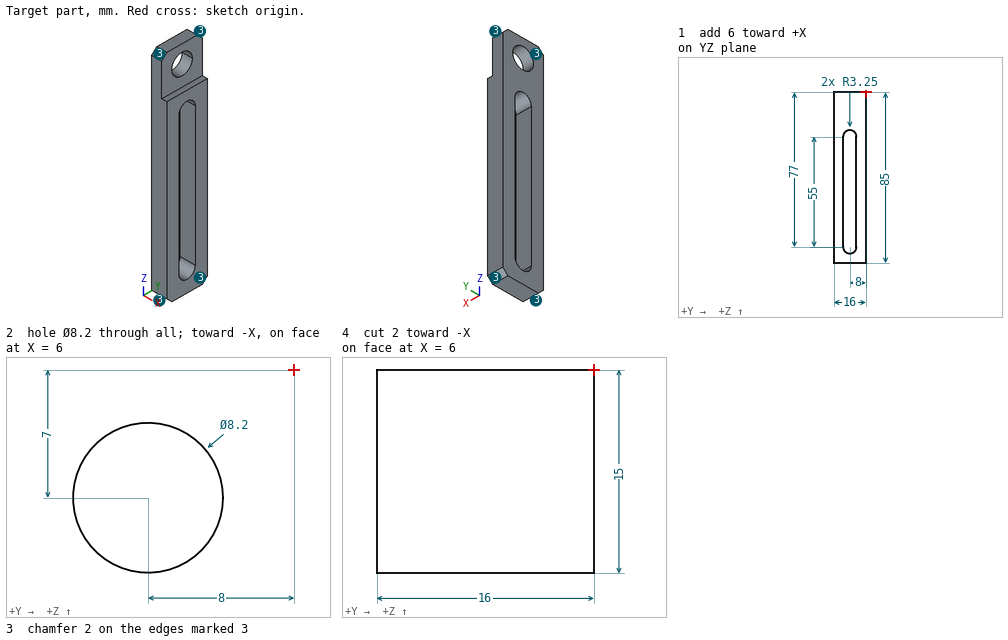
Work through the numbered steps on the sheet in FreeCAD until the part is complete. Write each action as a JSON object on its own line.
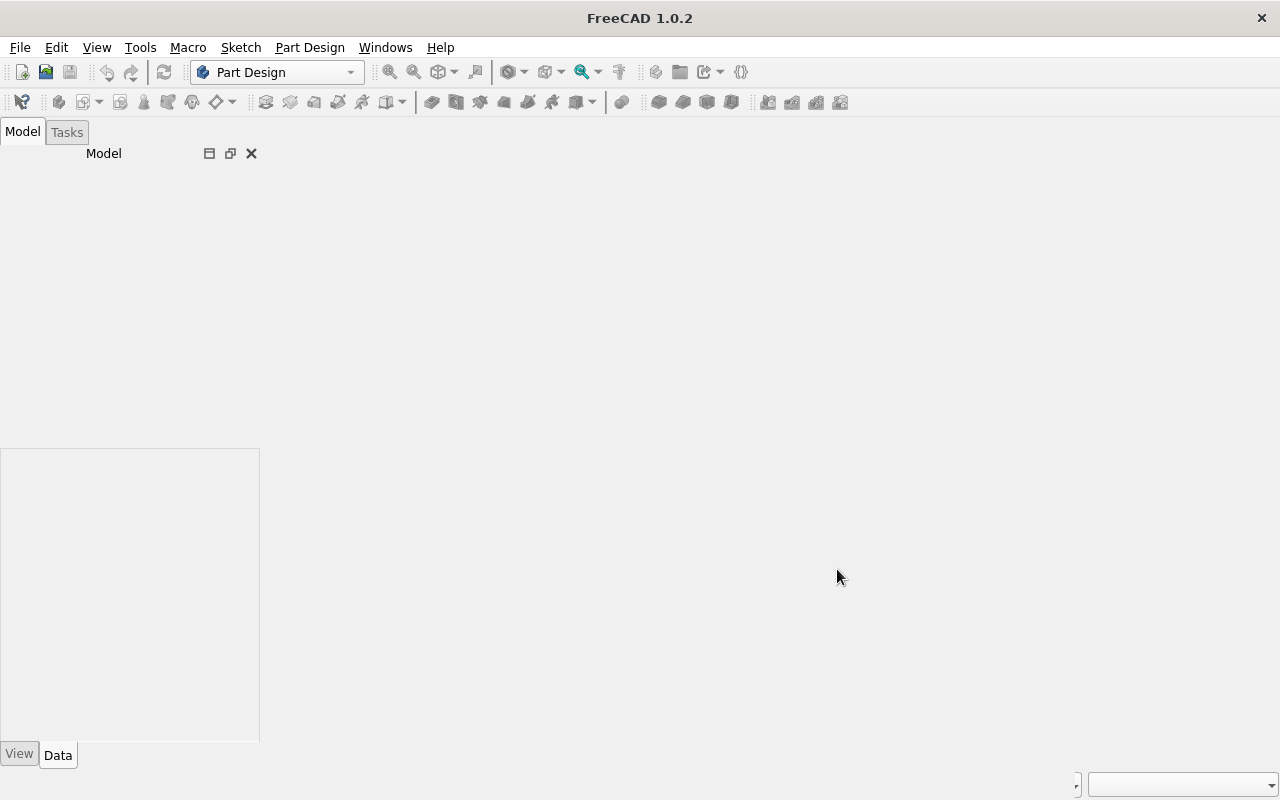
{"action": "key", "text": "ctrl+n"}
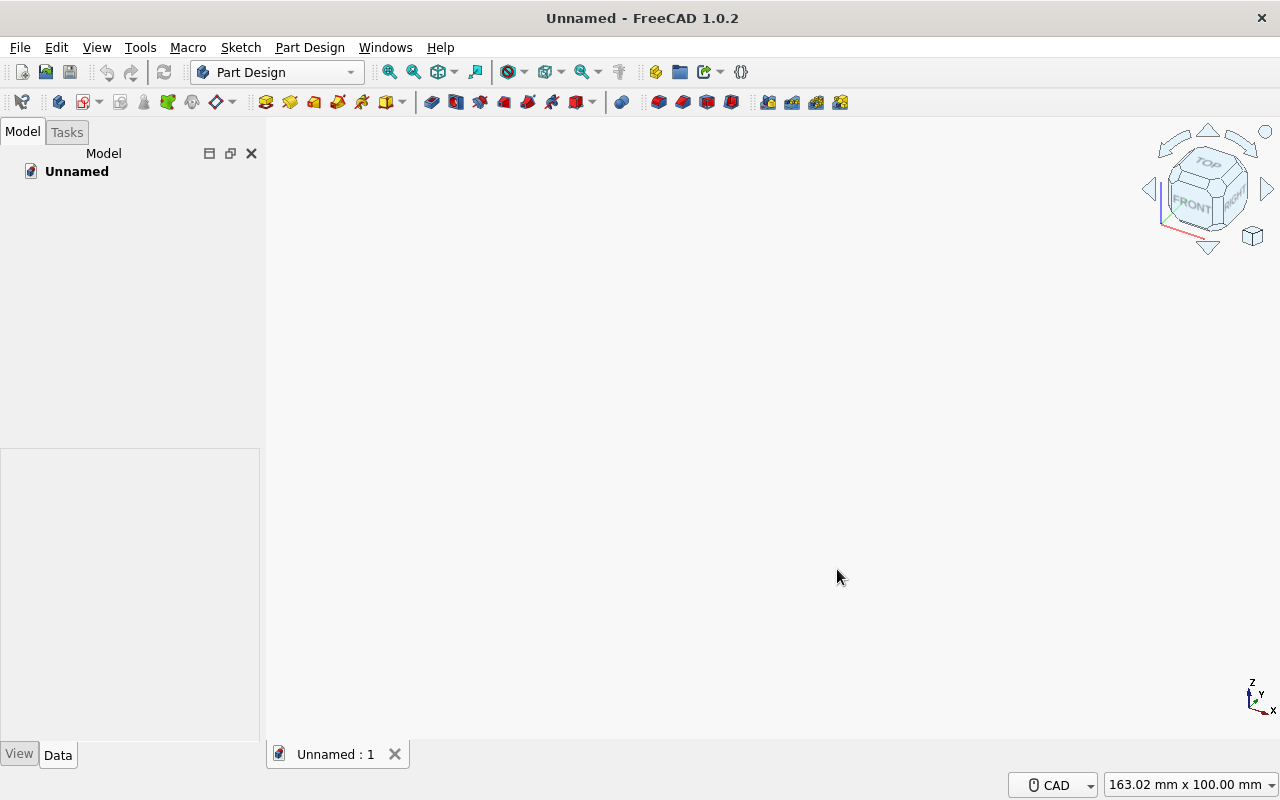
{"action": "left_click", "coordinate": [84, 102]}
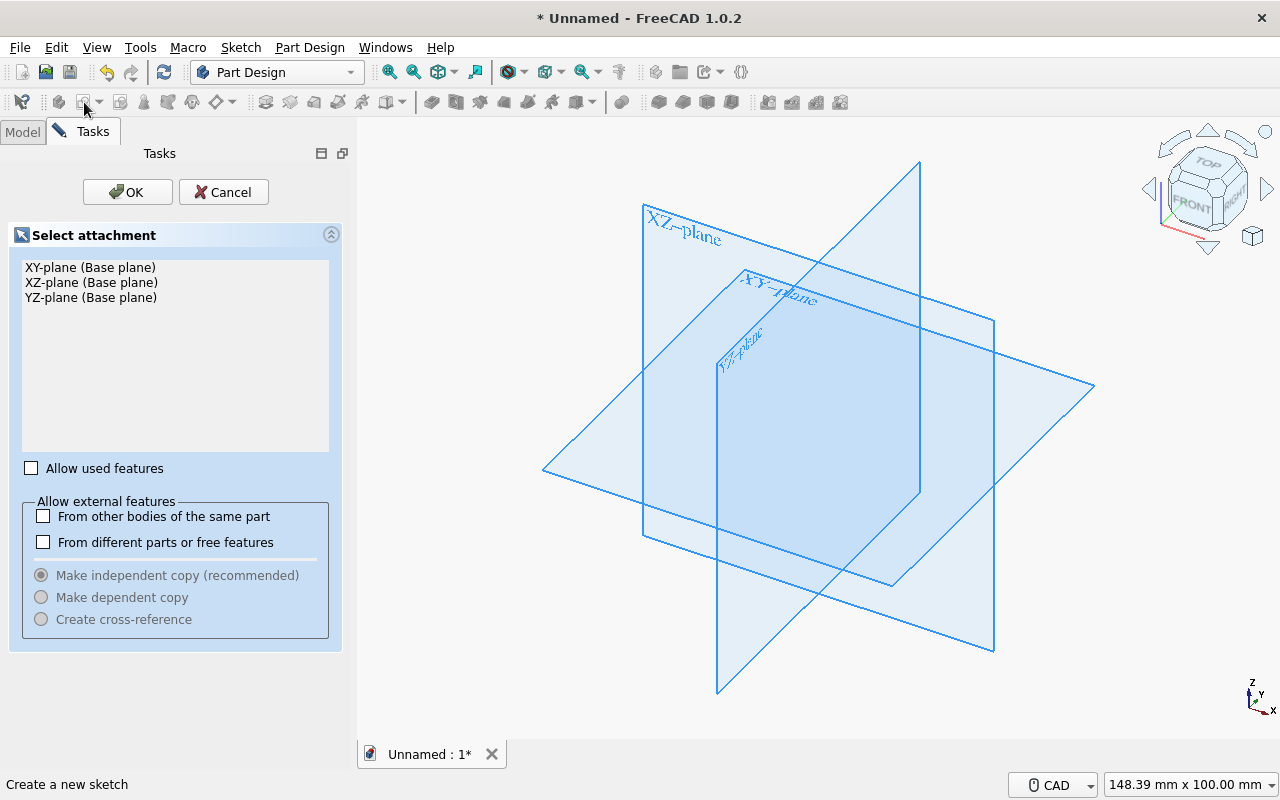
{"action": "left_click", "coordinate": [82, 298]}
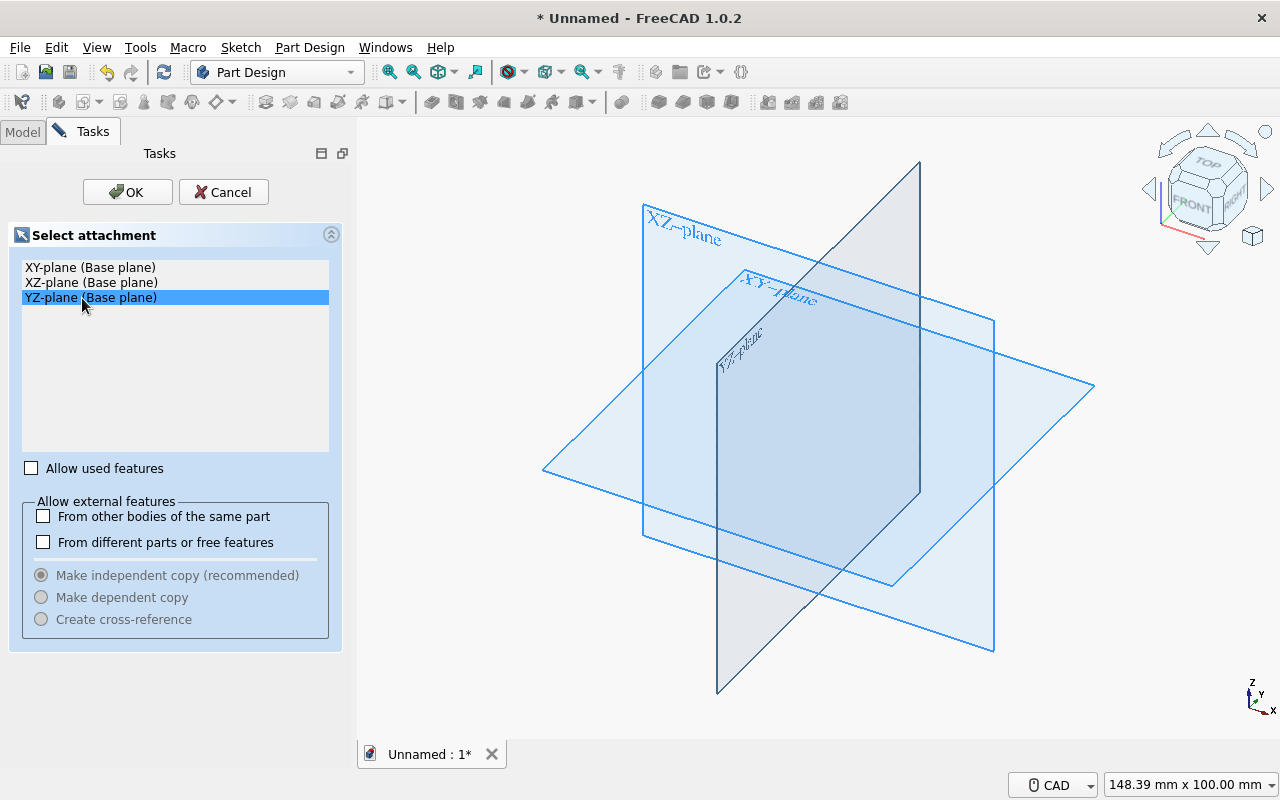
{"action": "left_click", "coordinate": [128, 192]}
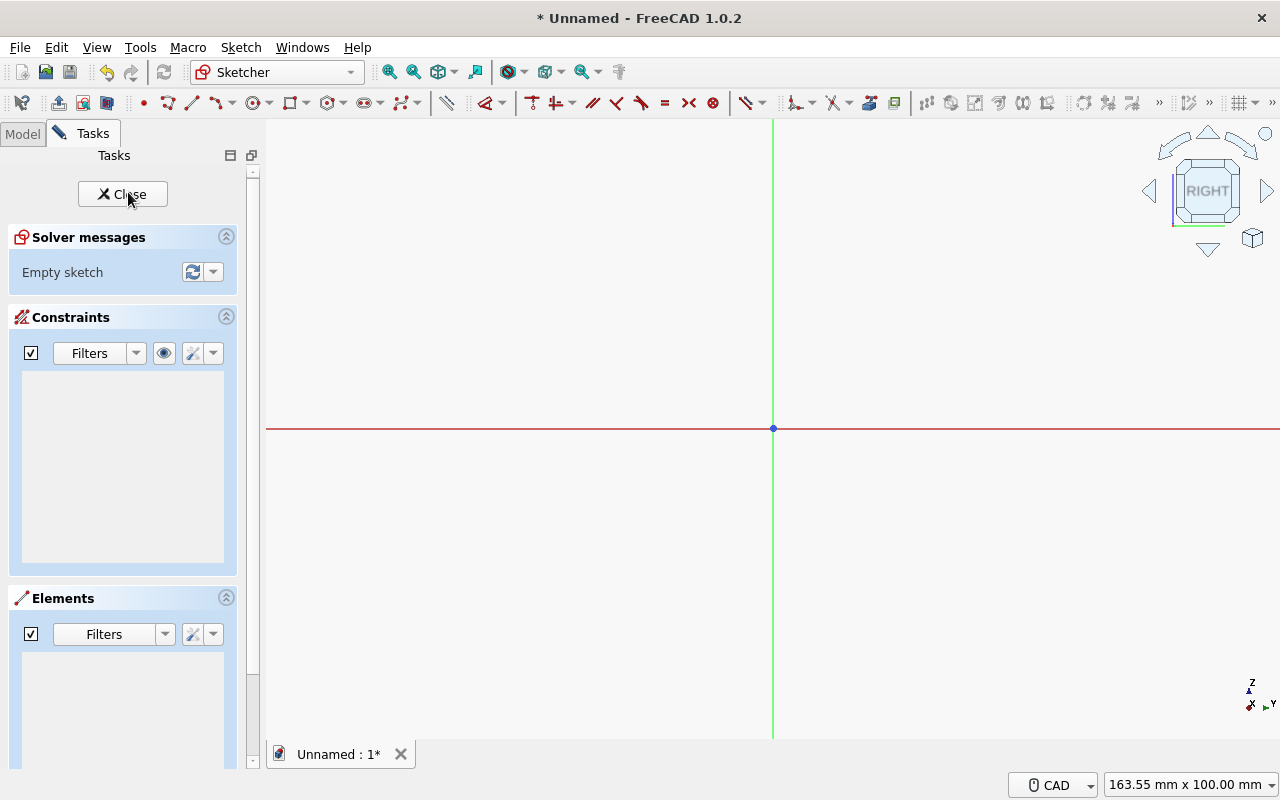
{"action": "scroll", "coordinate": [682, 147], "scroll_direction": "down", "scroll_amount": 3}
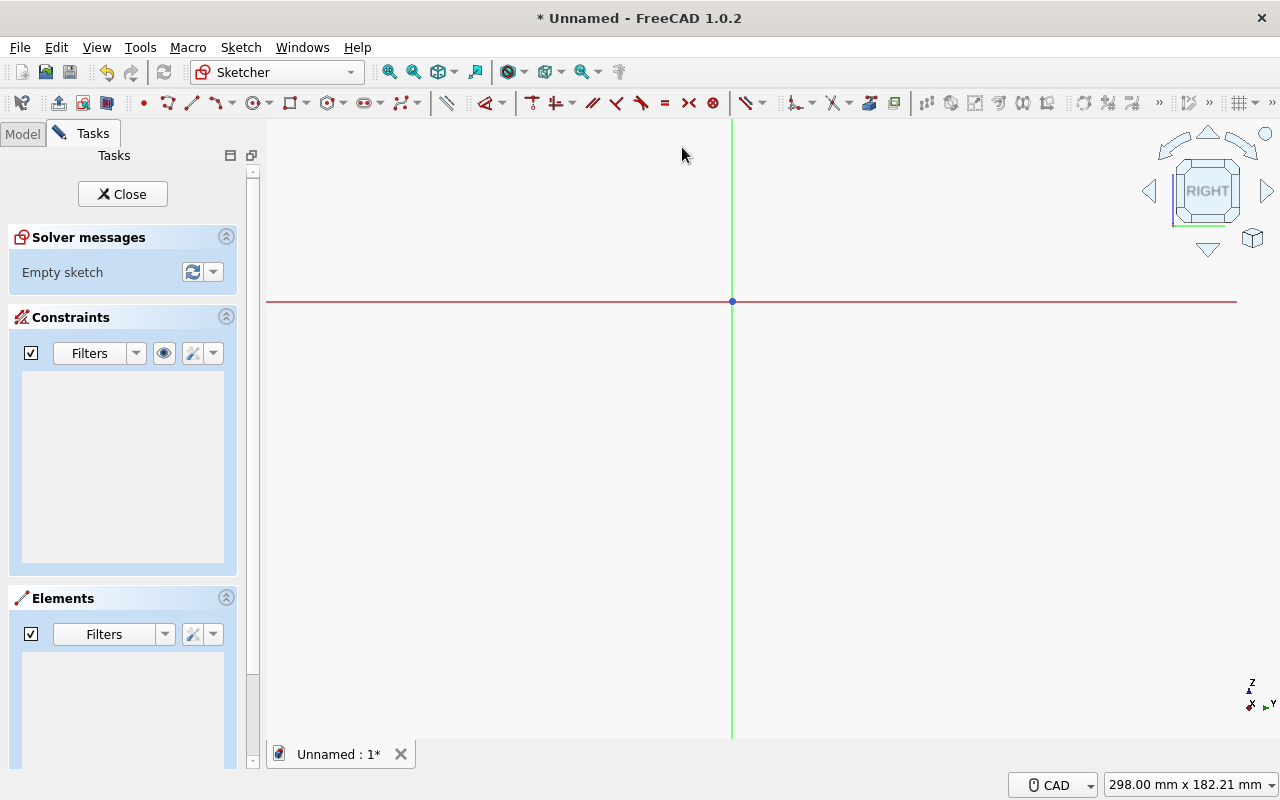
{"action": "scroll", "coordinate": [706, 482], "scroll_direction": "up", "scroll_amount": 2}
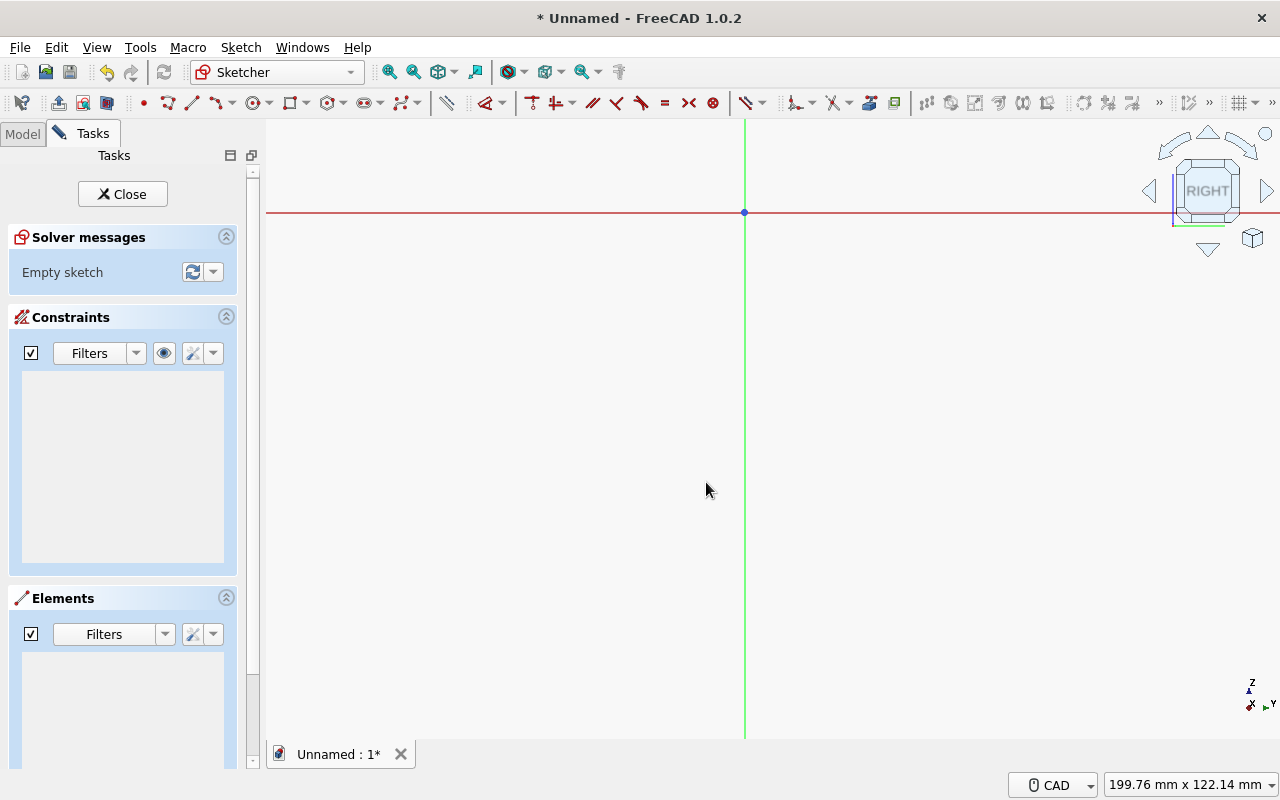
{"action": "left_click", "coordinate": [290, 104]}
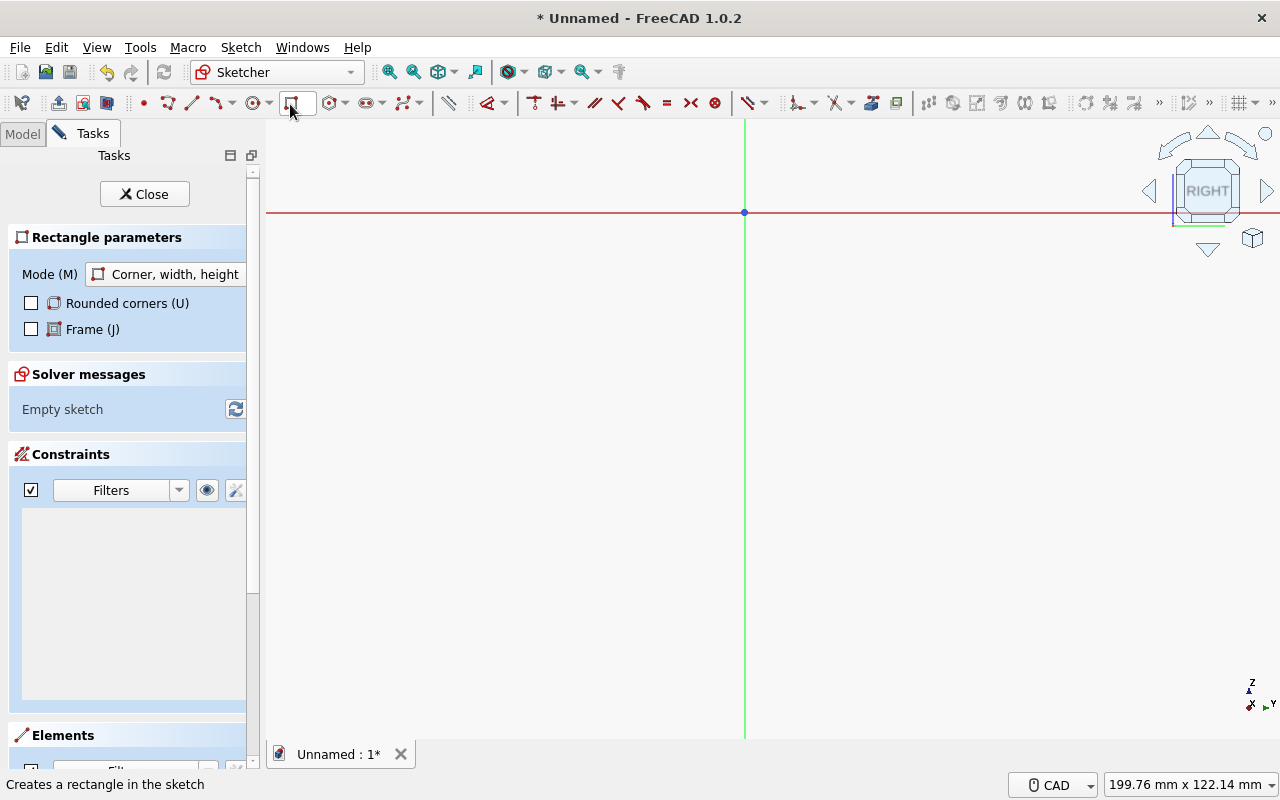
{"action": "left_click", "coordinate": [745, 213]}
{"action": "mouse_move", "coordinate": [664, 644]}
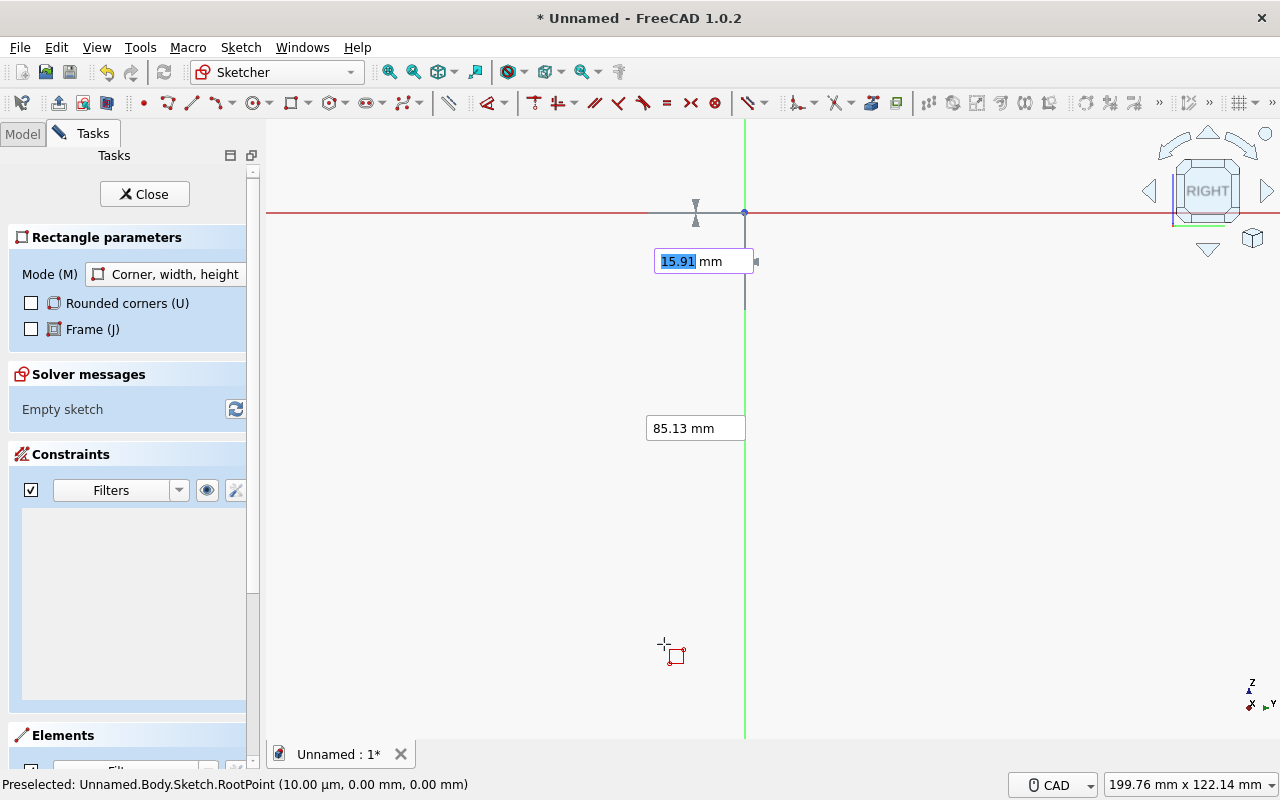
{"action": "type", "text": "16"}
{"action": "key", "text": "Tab"}
{"action": "type", "text": "85"}
{"action": "key", "text": "Return"}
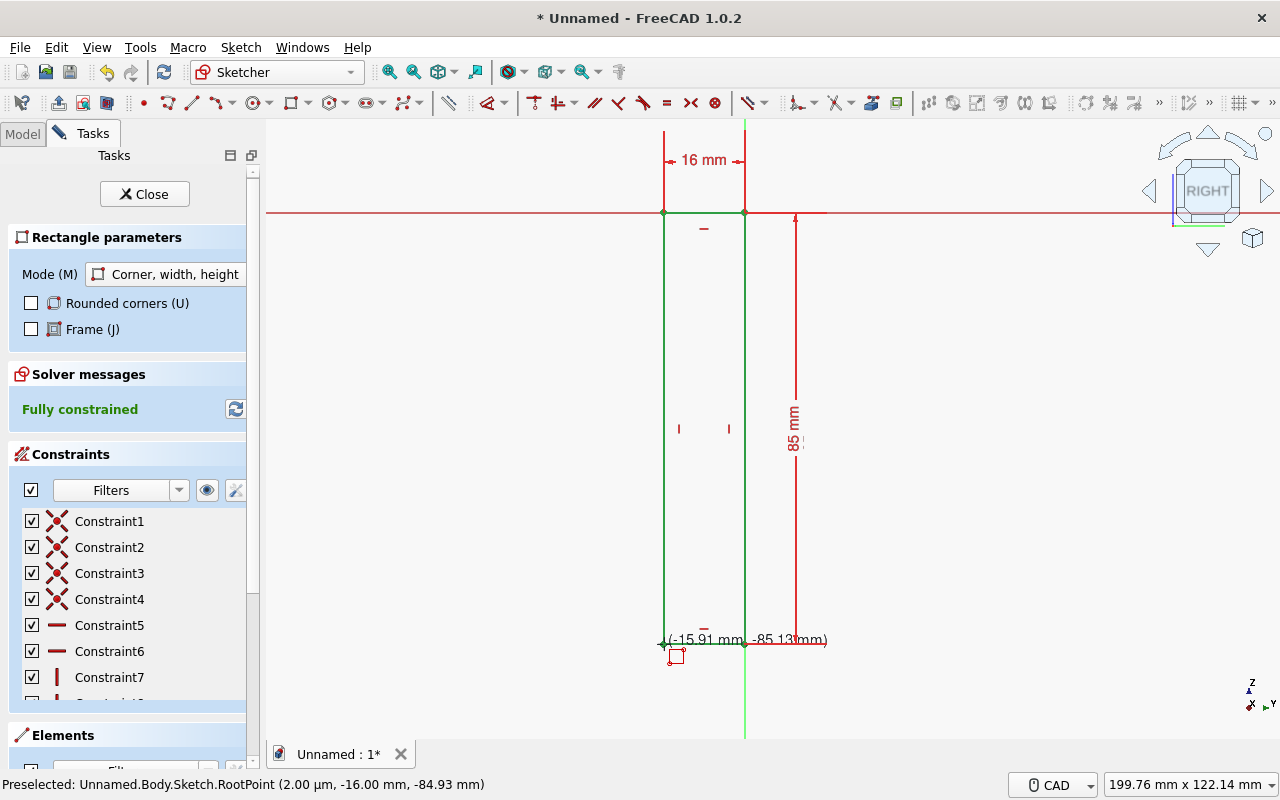
{"action": "left_click", "coordinate": [366, 104]}